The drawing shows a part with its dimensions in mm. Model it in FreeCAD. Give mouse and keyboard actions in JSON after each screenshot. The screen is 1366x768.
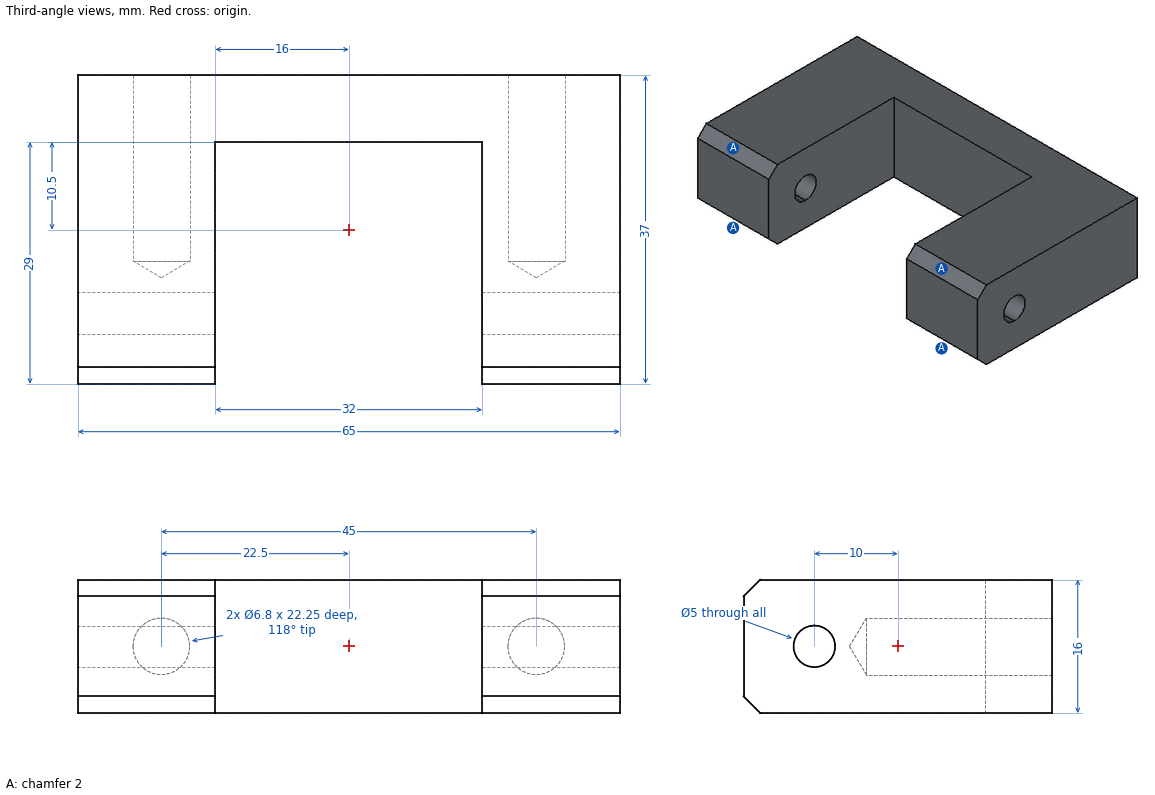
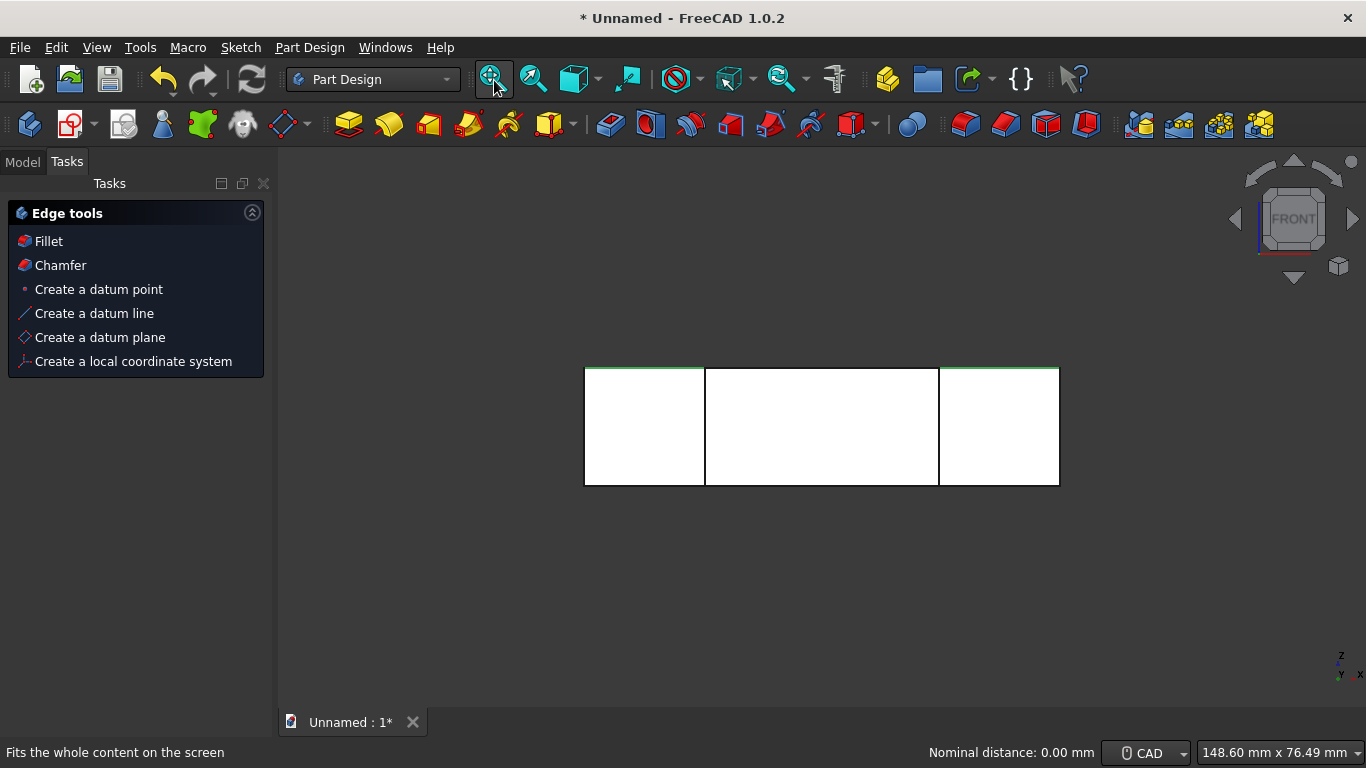
{"action": "left_click", "coordinate": [1000, 485], "text": "ctrl"}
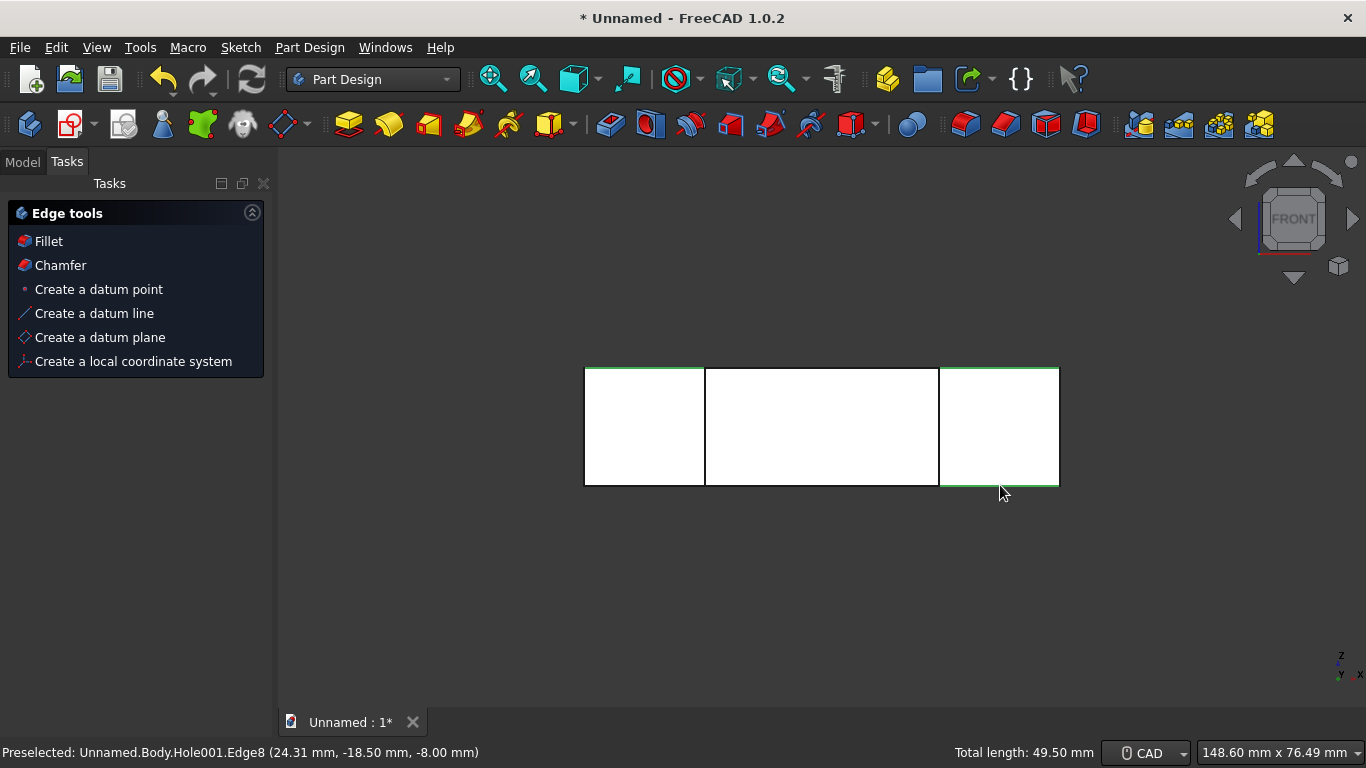
{"action": "left_click", "coordinate": [644, 485], "text": "ctrl"}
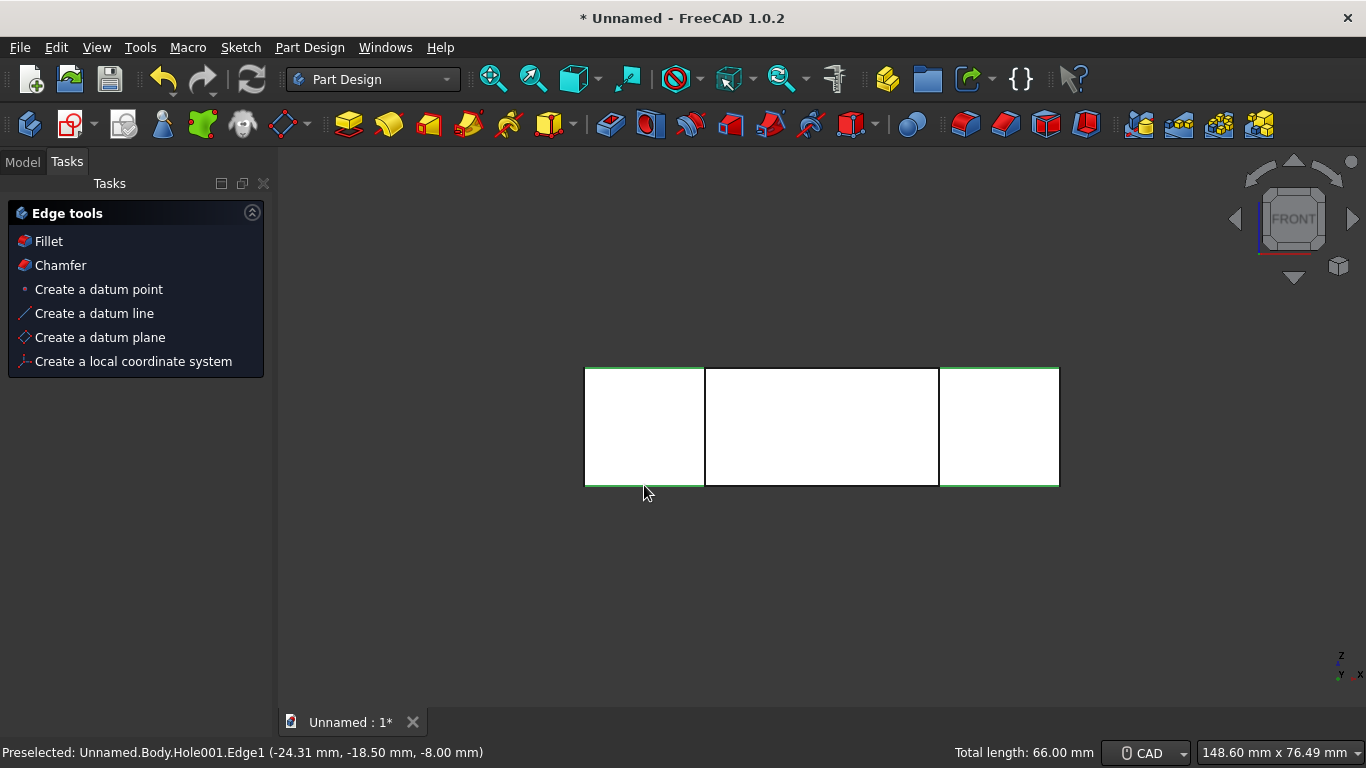
{"action": "left_click", "coordinate": [1006, 124]}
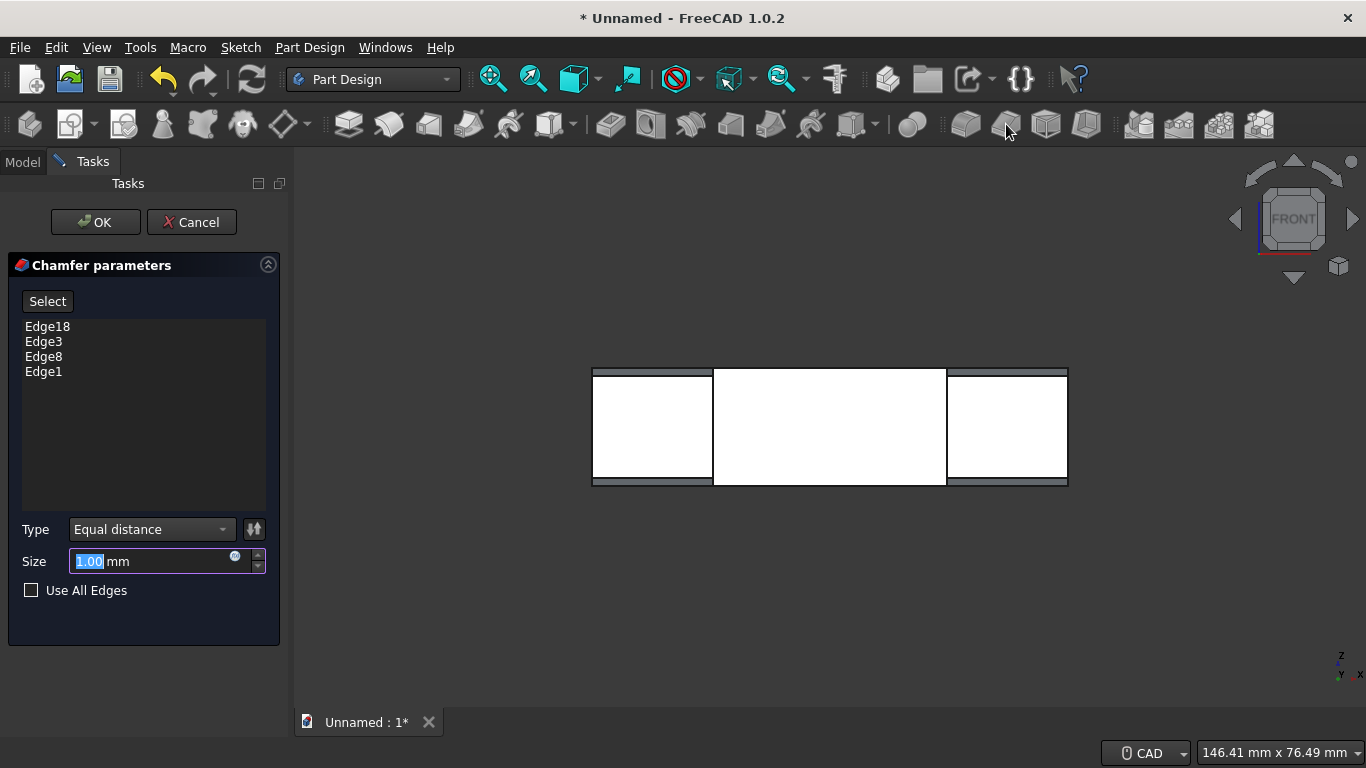
{"action": "type", "text": "2"}
{"action": "key", "text": "Tab"}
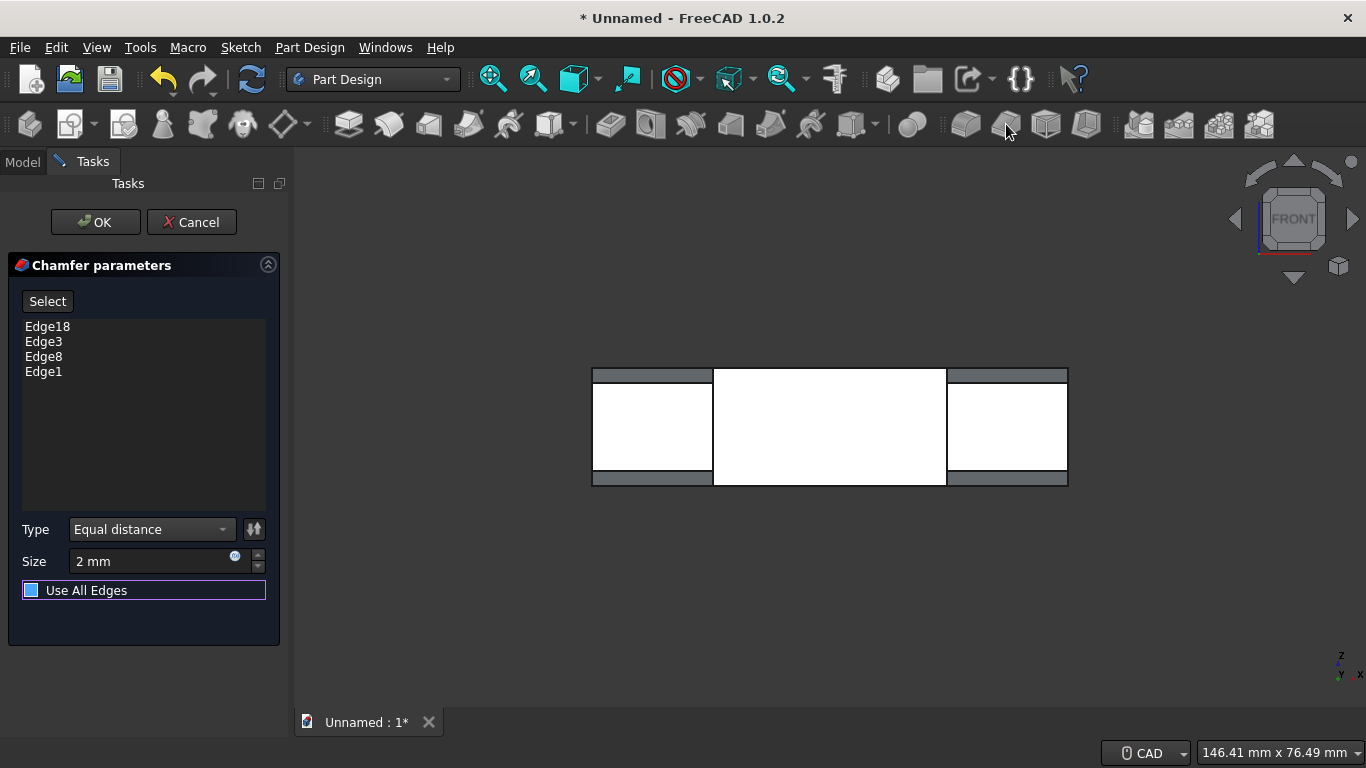
{"action": "left_click", "coordinate": [96, 222]}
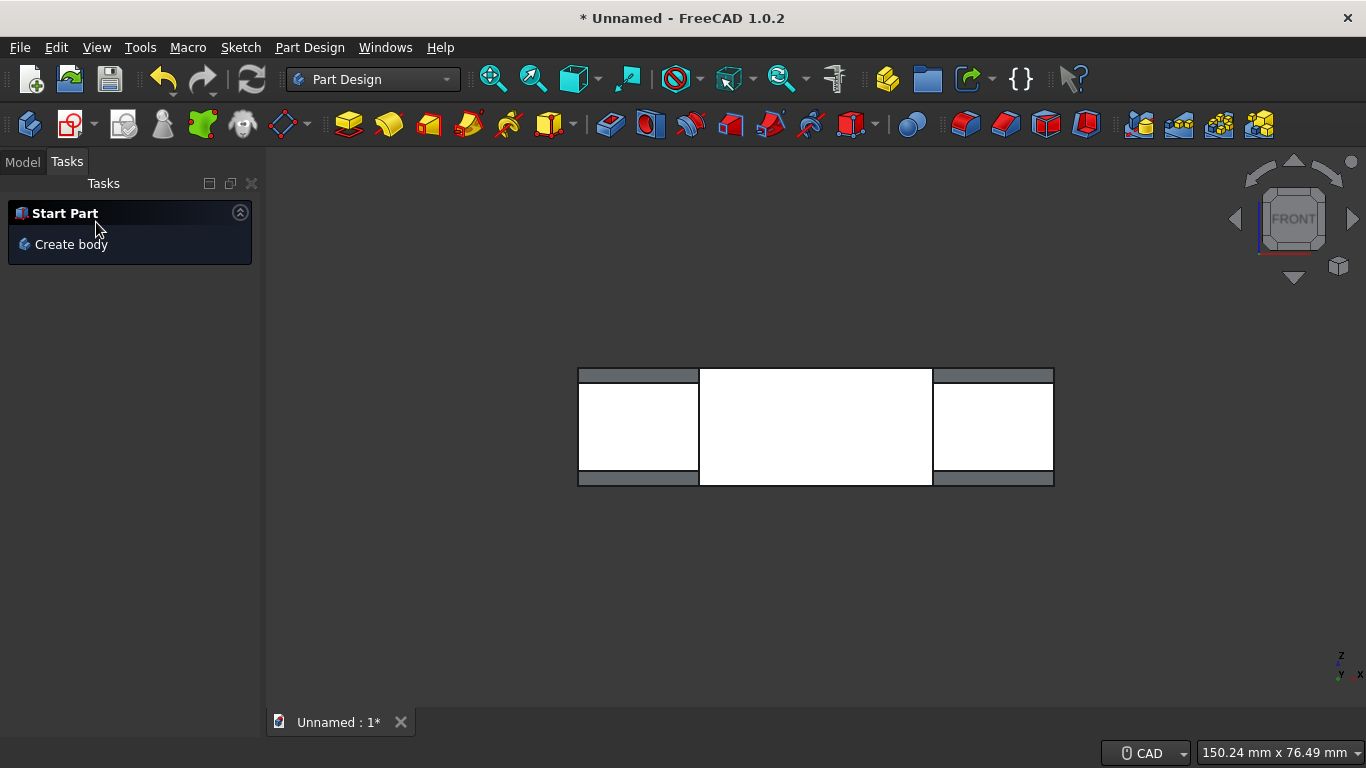
{"action": "key", "text": "0"}